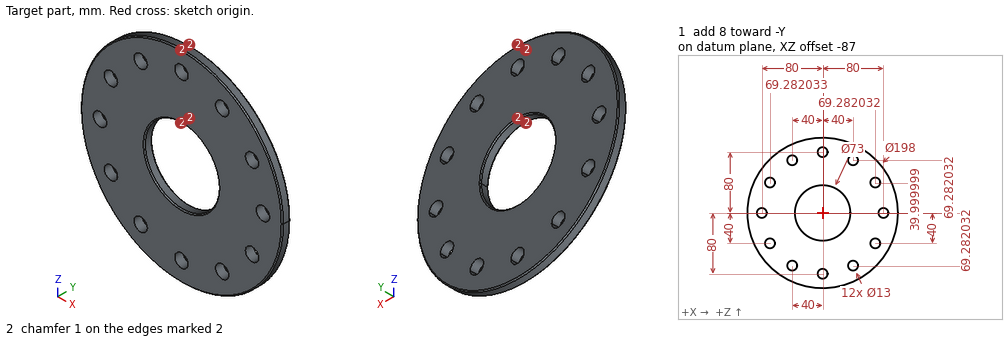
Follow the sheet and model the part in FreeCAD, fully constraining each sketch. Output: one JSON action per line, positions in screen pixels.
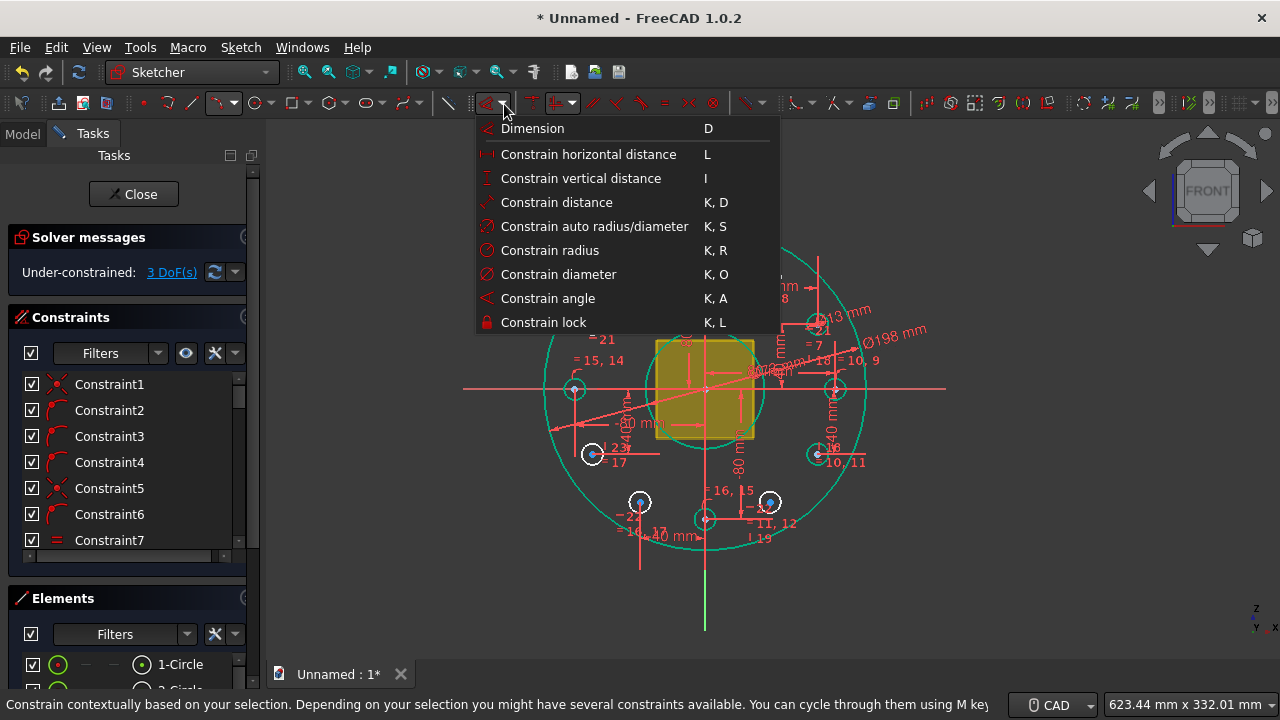
{"action": "left_click", "coordinate": [628, 178]}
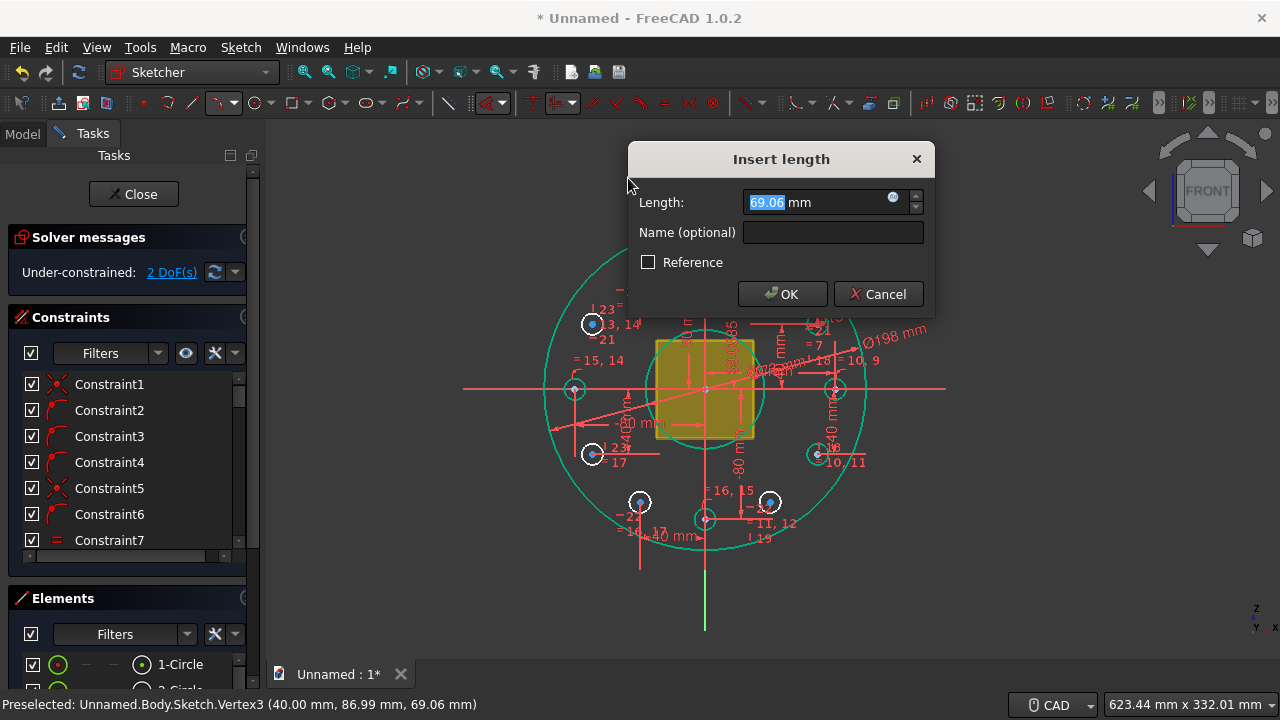
{"action": "type", "text": "69.282032"}
{"action": "key", "text": "Return"}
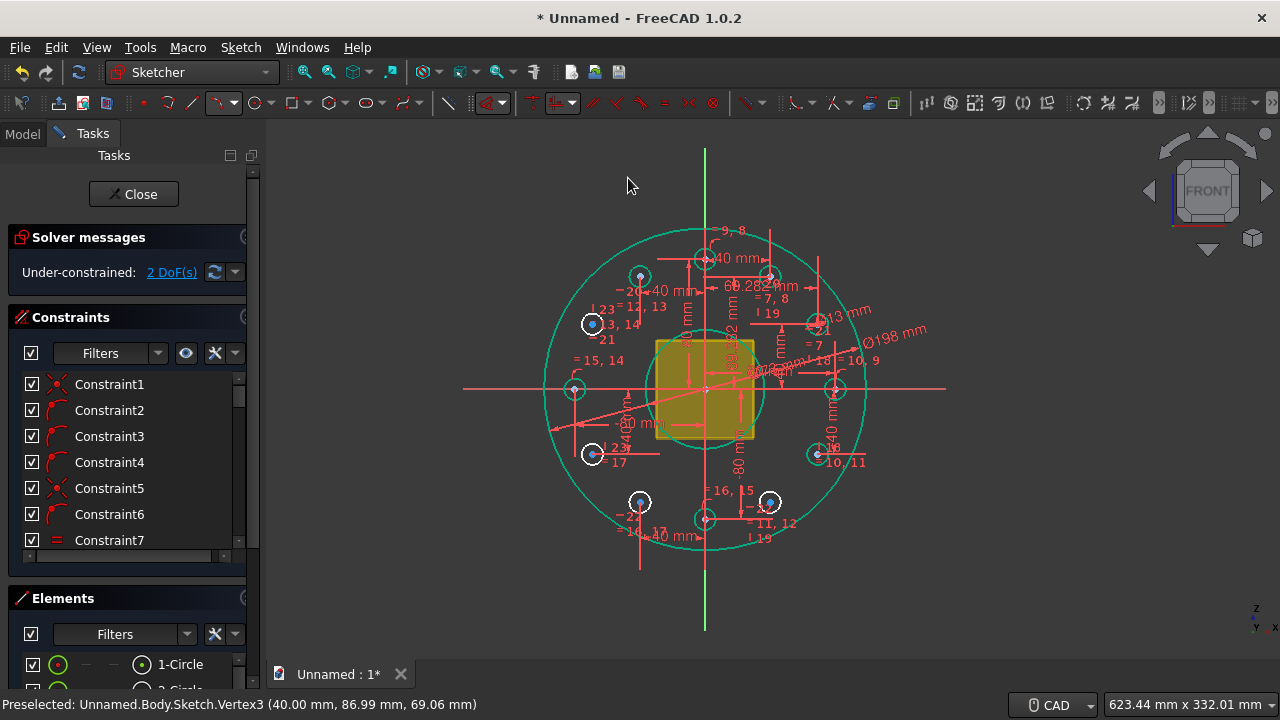
{"action": "left_click", "coordinate": [770, 502]}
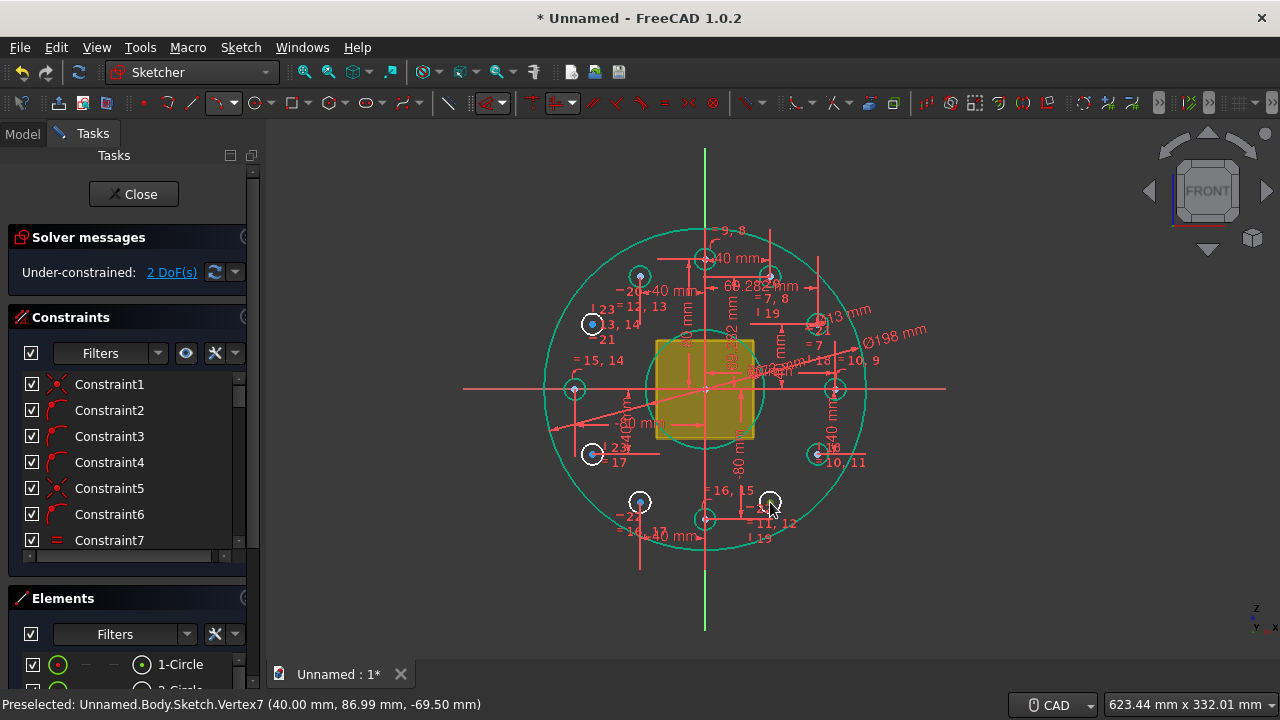
{"action": "key", "text": "i"}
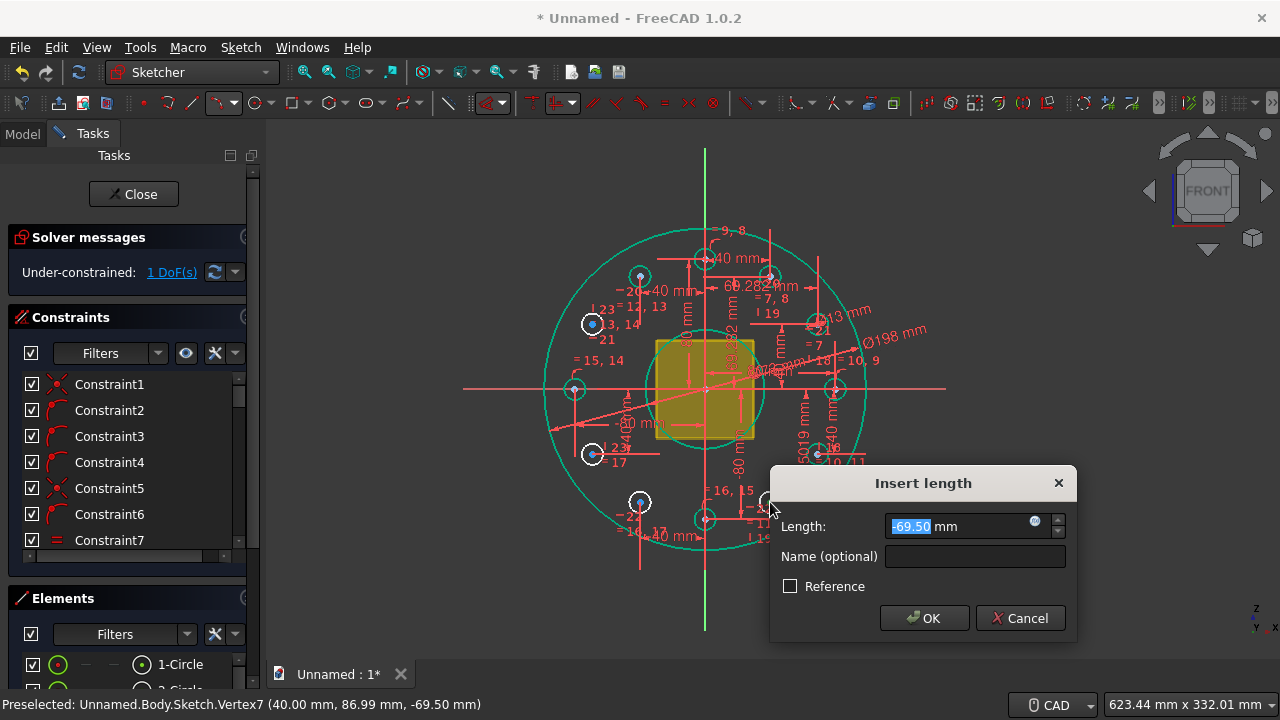
{"action": "type", "text": "-69.282032"}
{"action": "key", "text": "Return"}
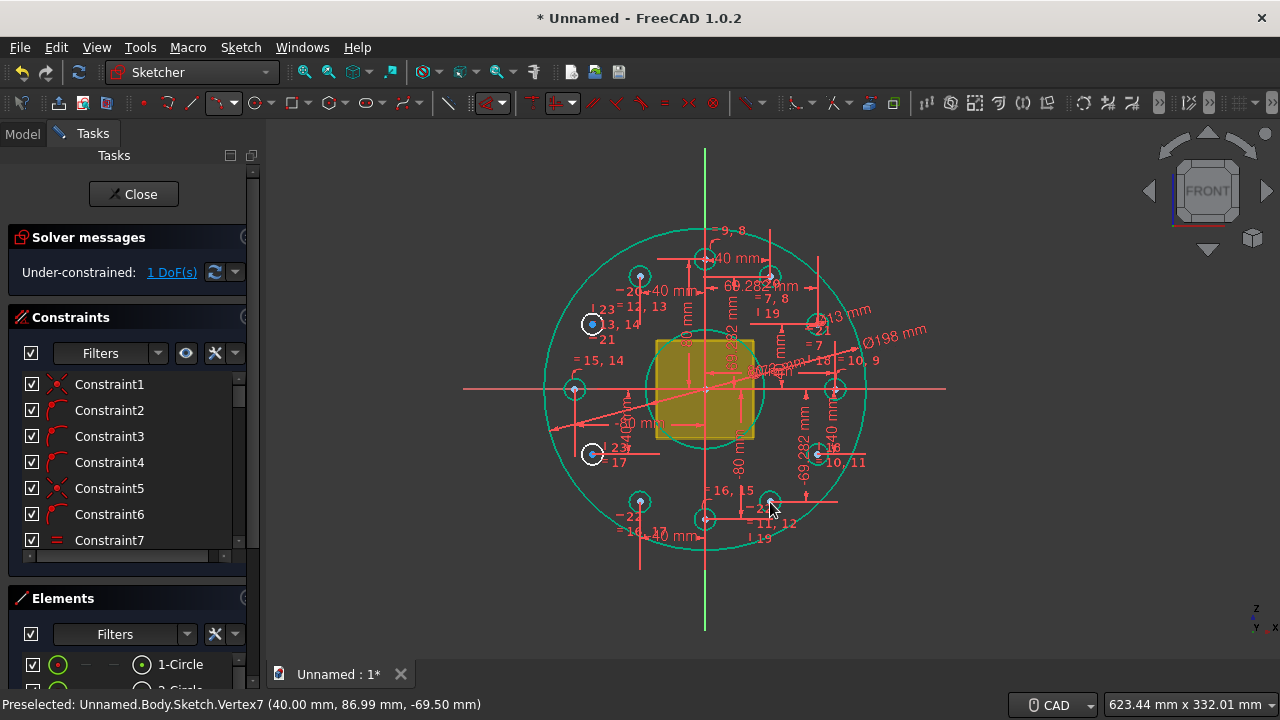
{"action": "left_click", "coordinate": [592, 324]}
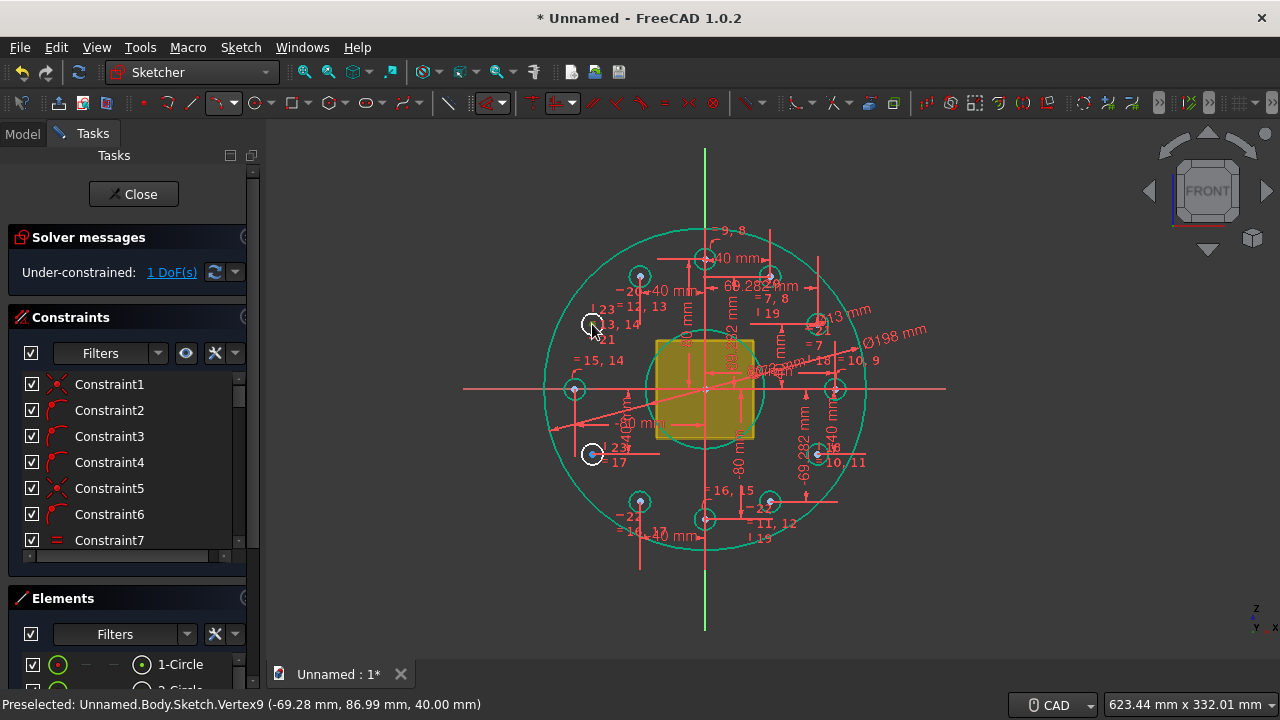
{"action": "key", "text": "l"}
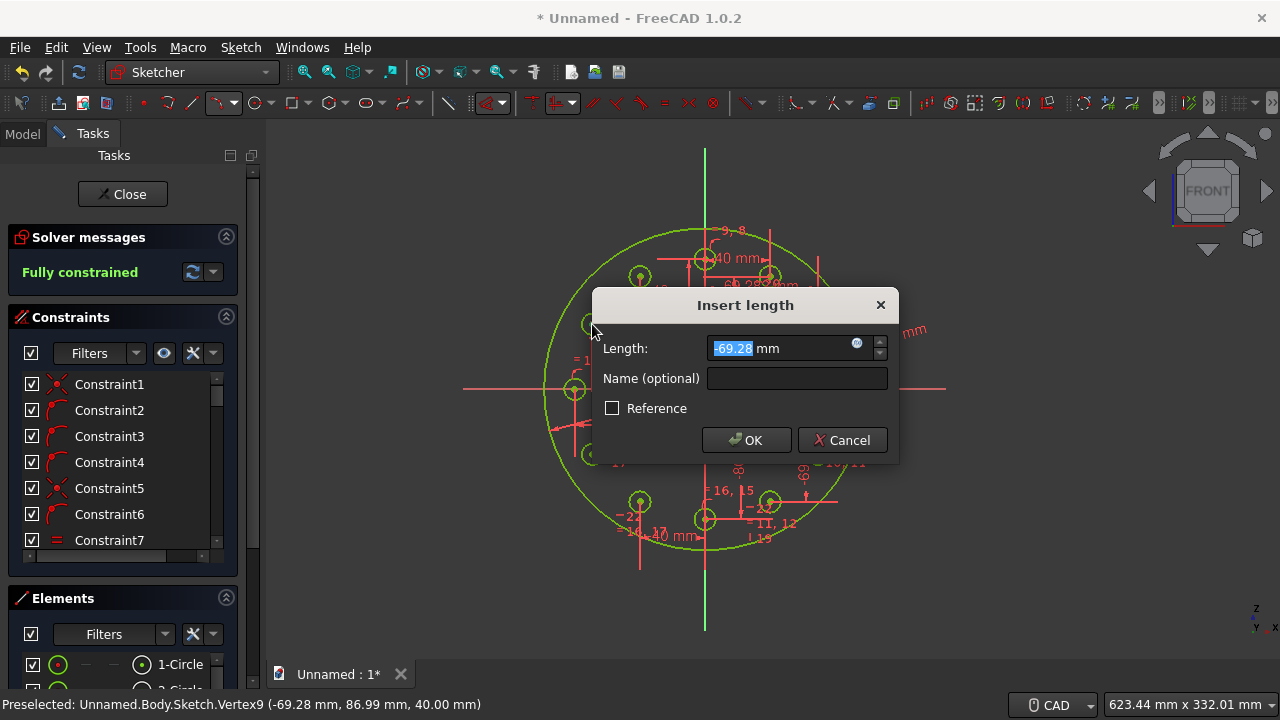
{"action": "type", "text": "-69.282033"}
{"action": "key", "text": "Return"}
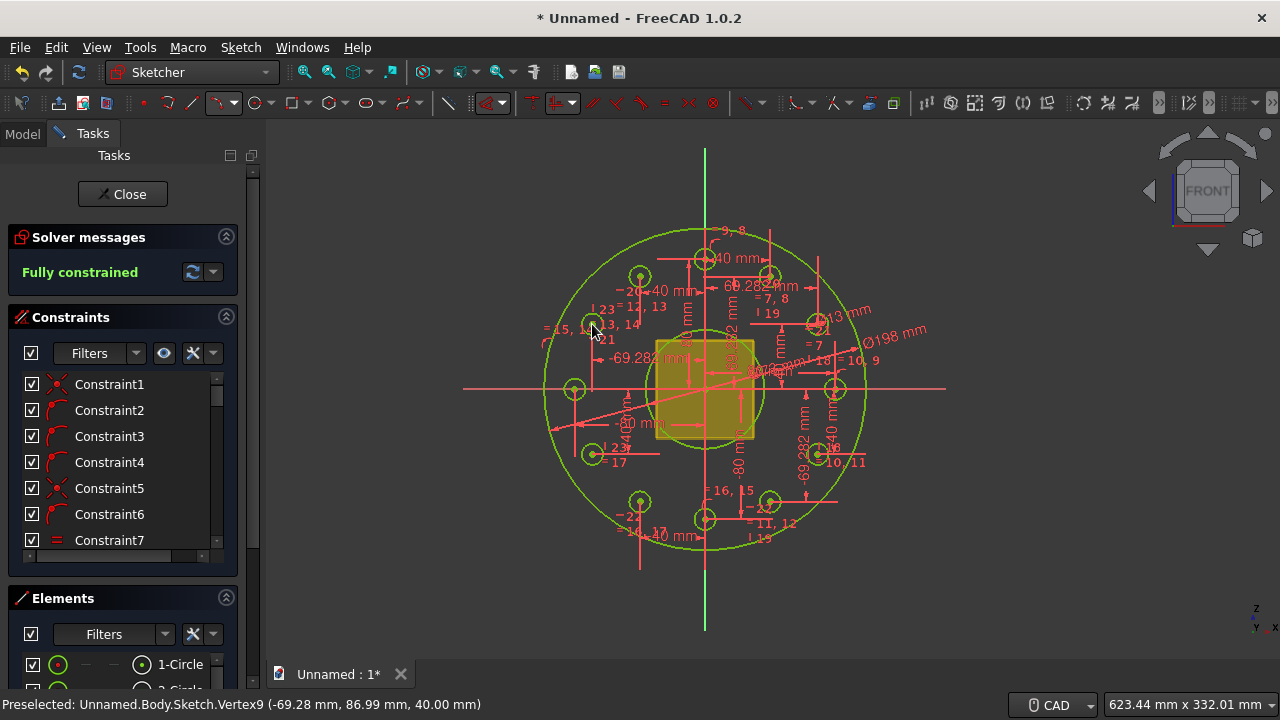
{"action": "left_click", "coordinate": [123, 194]}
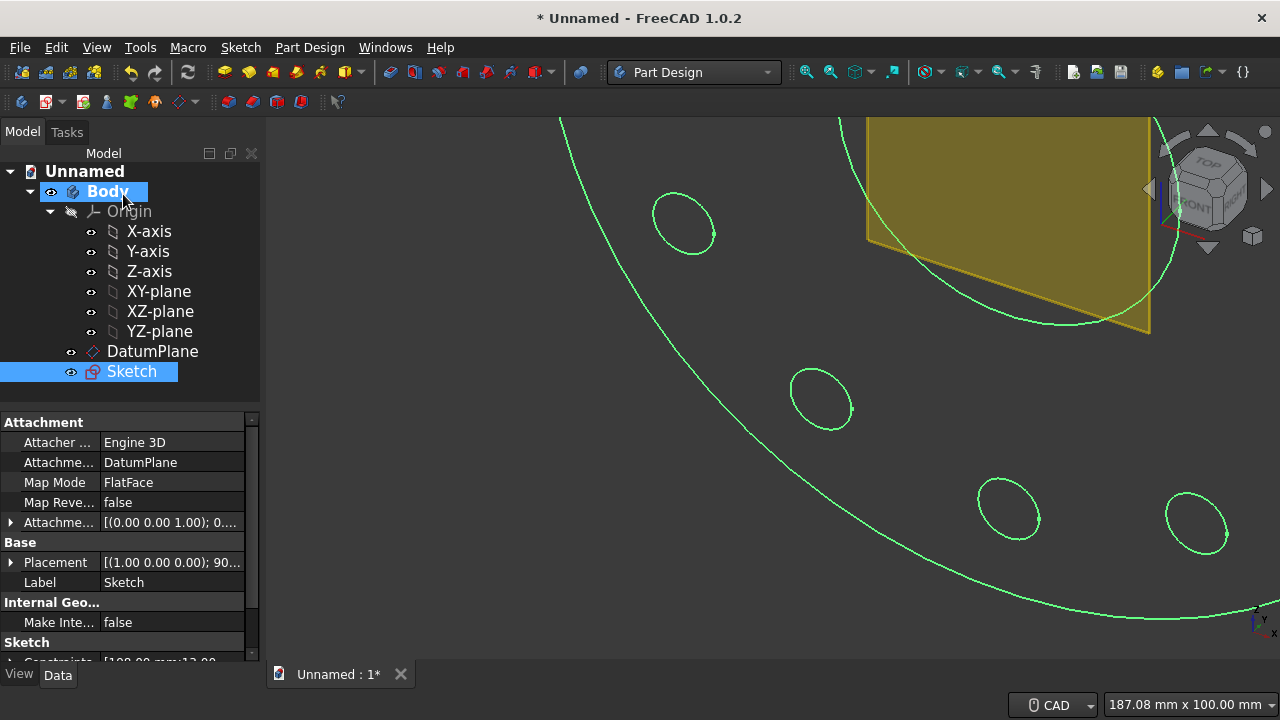
{"action": "left_click", "coordinate": [226, 72]}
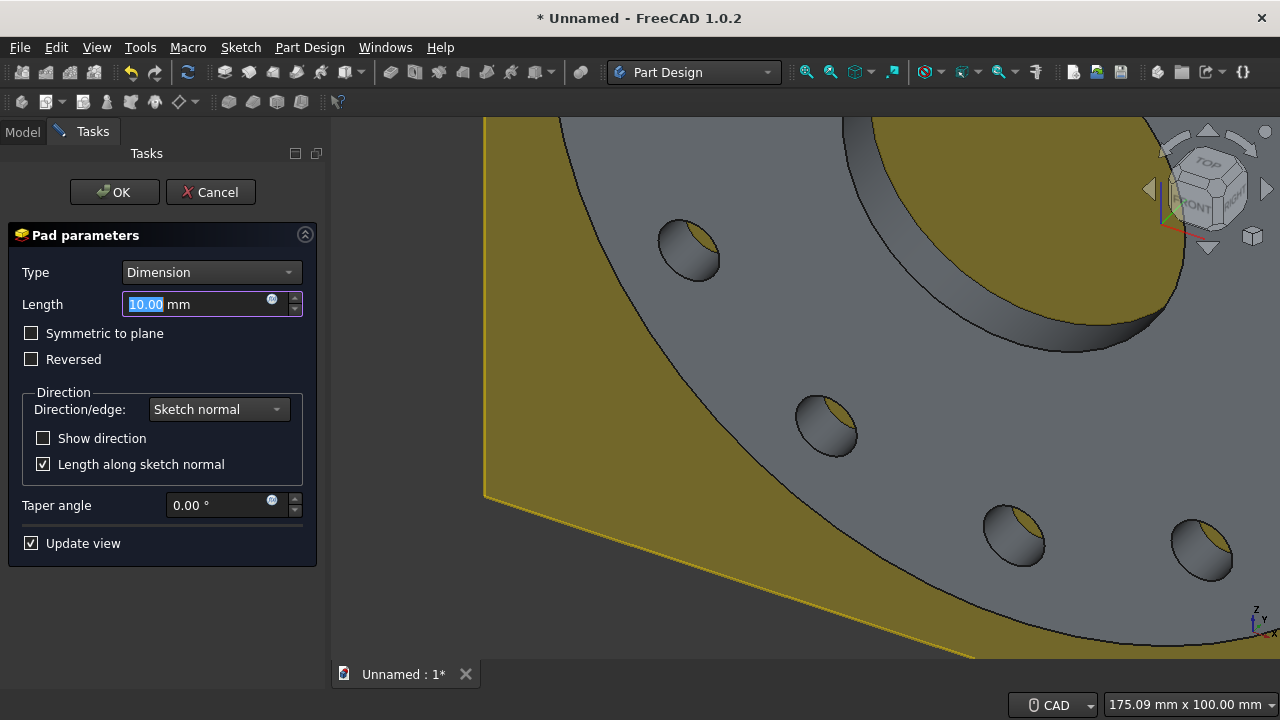
{"action": "type", "text": "8"}
{"action": "key", "text": "Tab"}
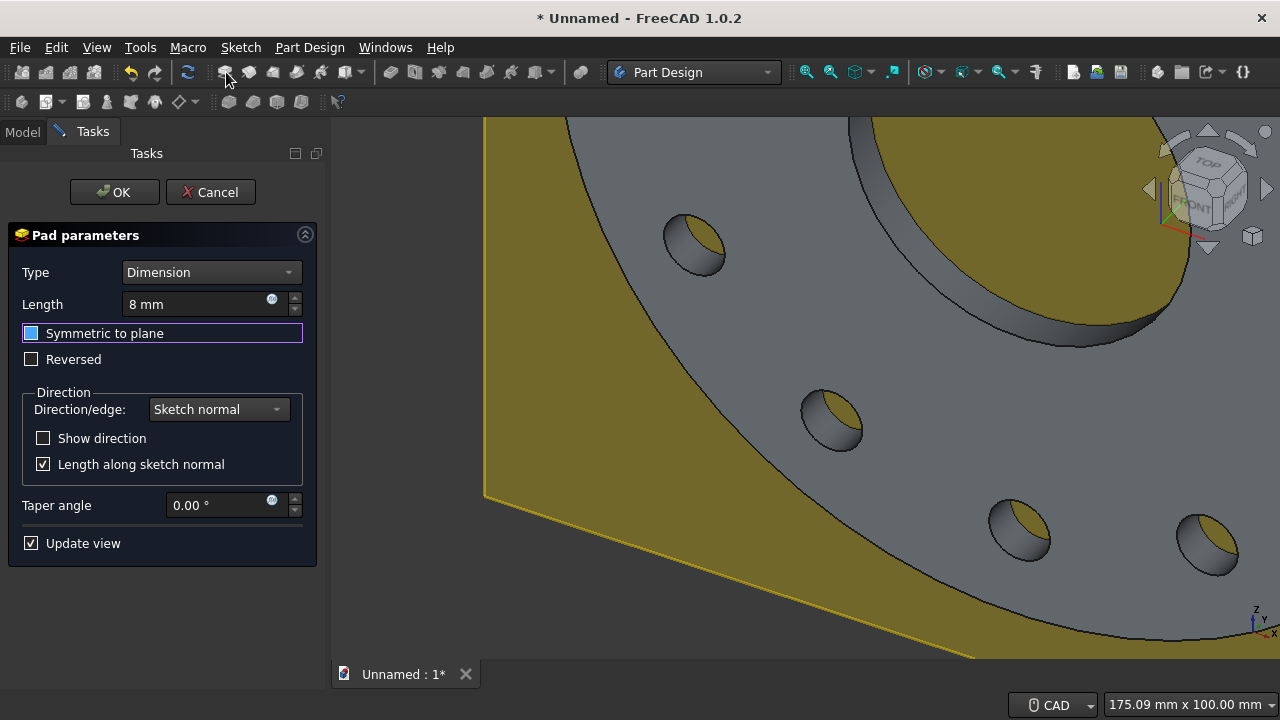
{"action": "left_click", "coordinate": [115, 192]}